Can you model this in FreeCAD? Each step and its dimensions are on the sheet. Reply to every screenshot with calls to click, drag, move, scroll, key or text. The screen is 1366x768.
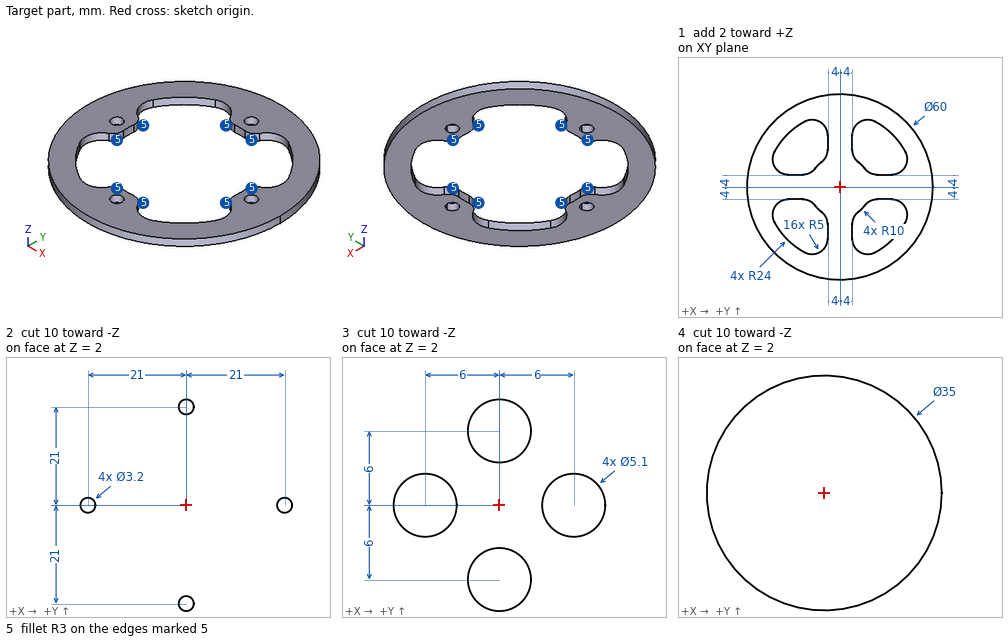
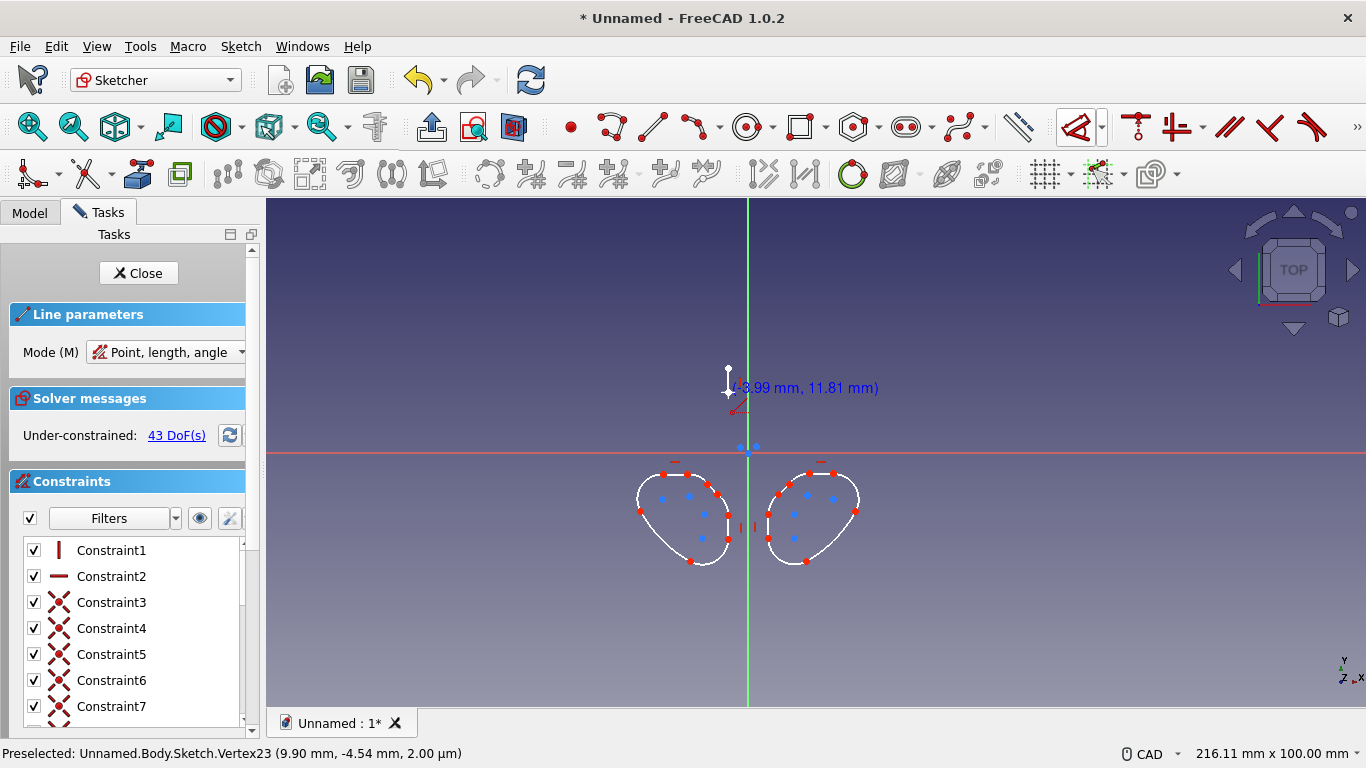
click(687, 433)
click(663, 433)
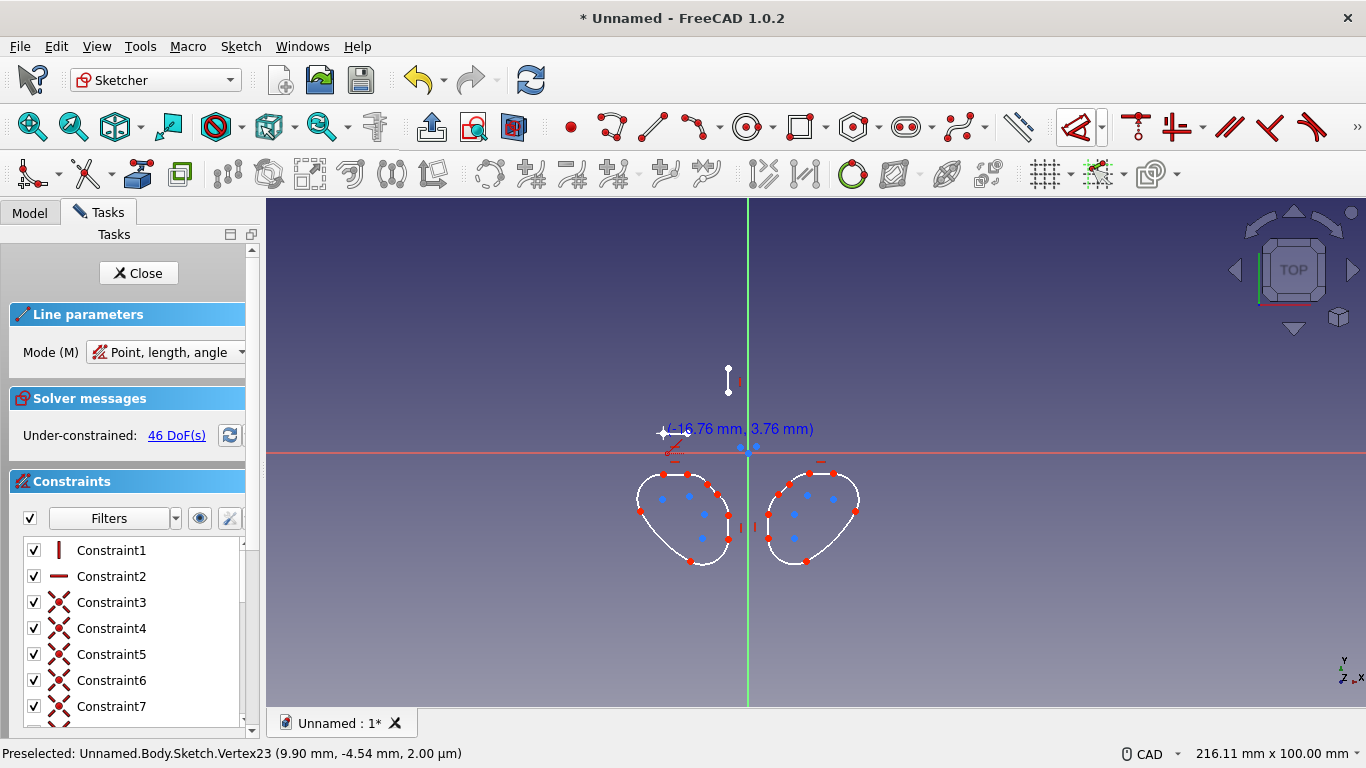
click(694, 128)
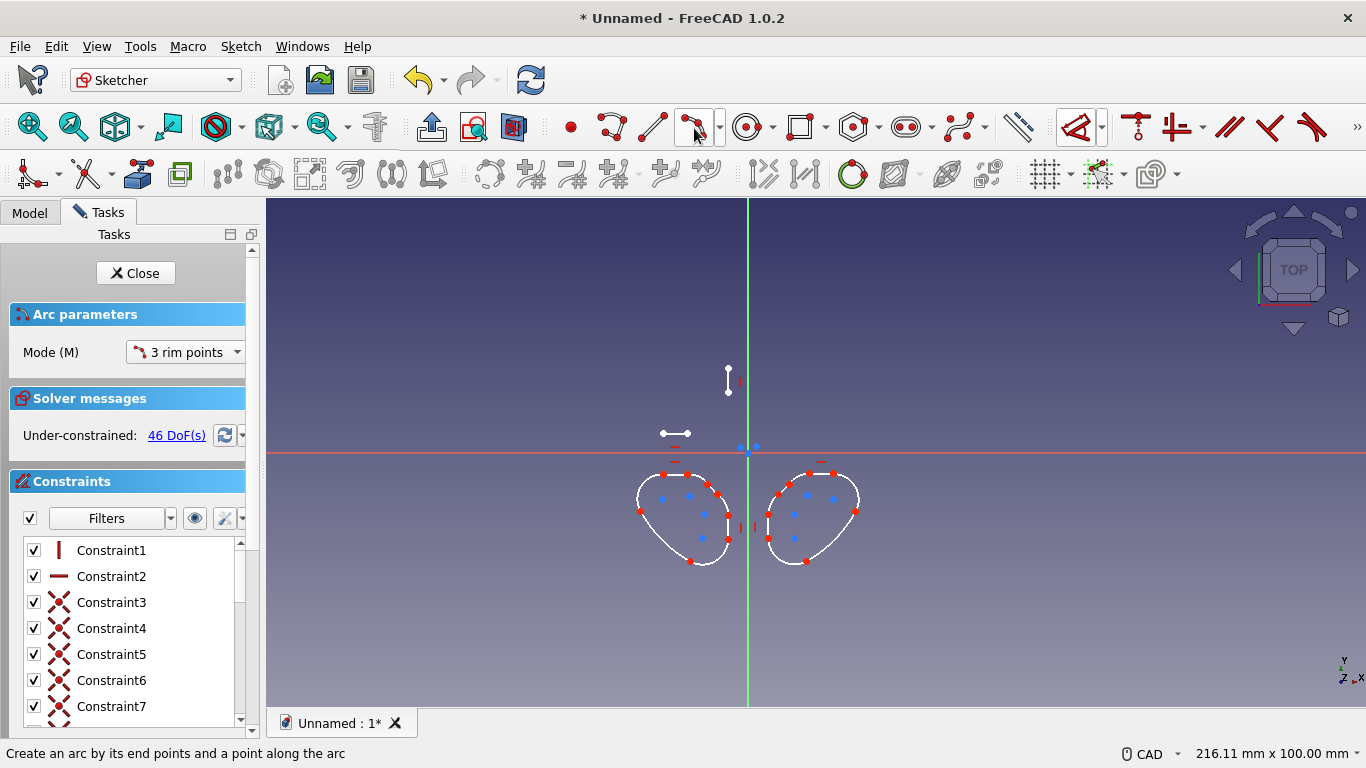
scroll(728, 392, up, 2)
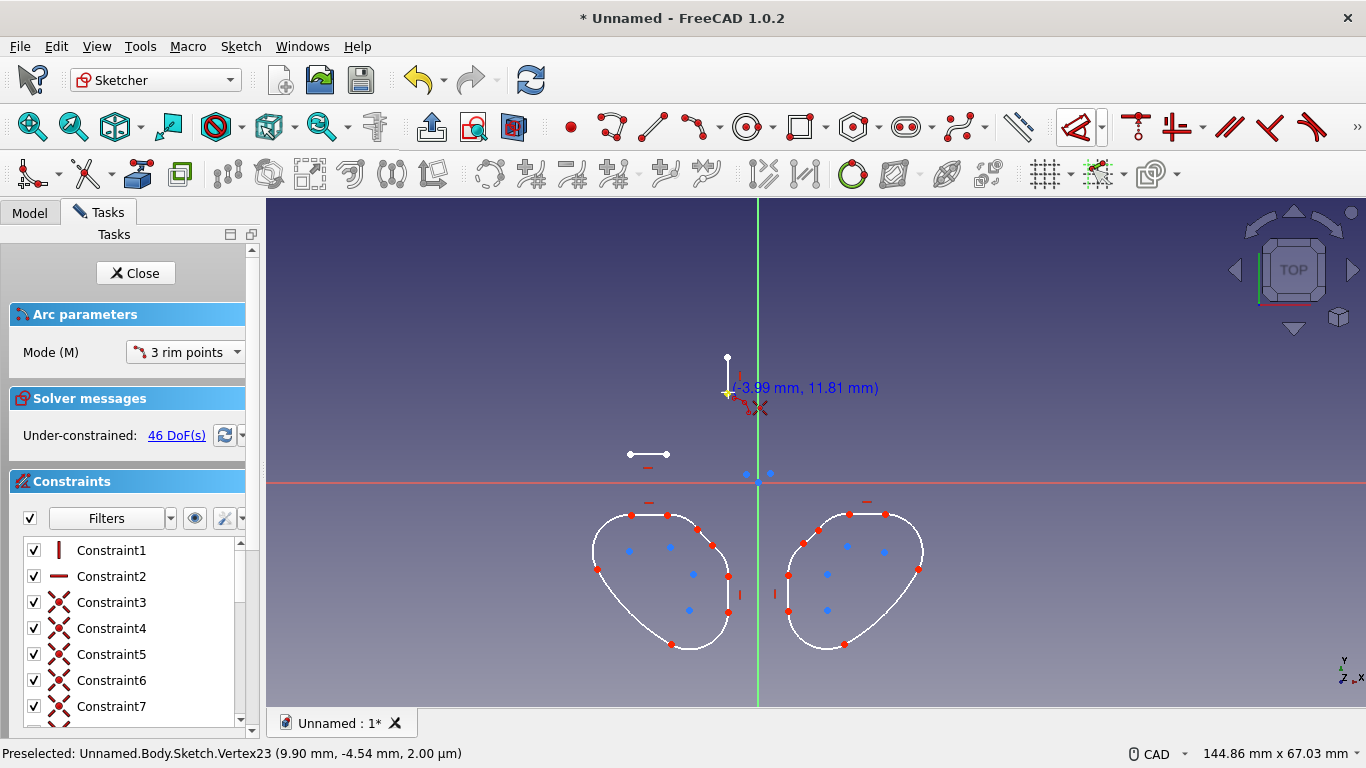
click(728, 393)
click(712, 422)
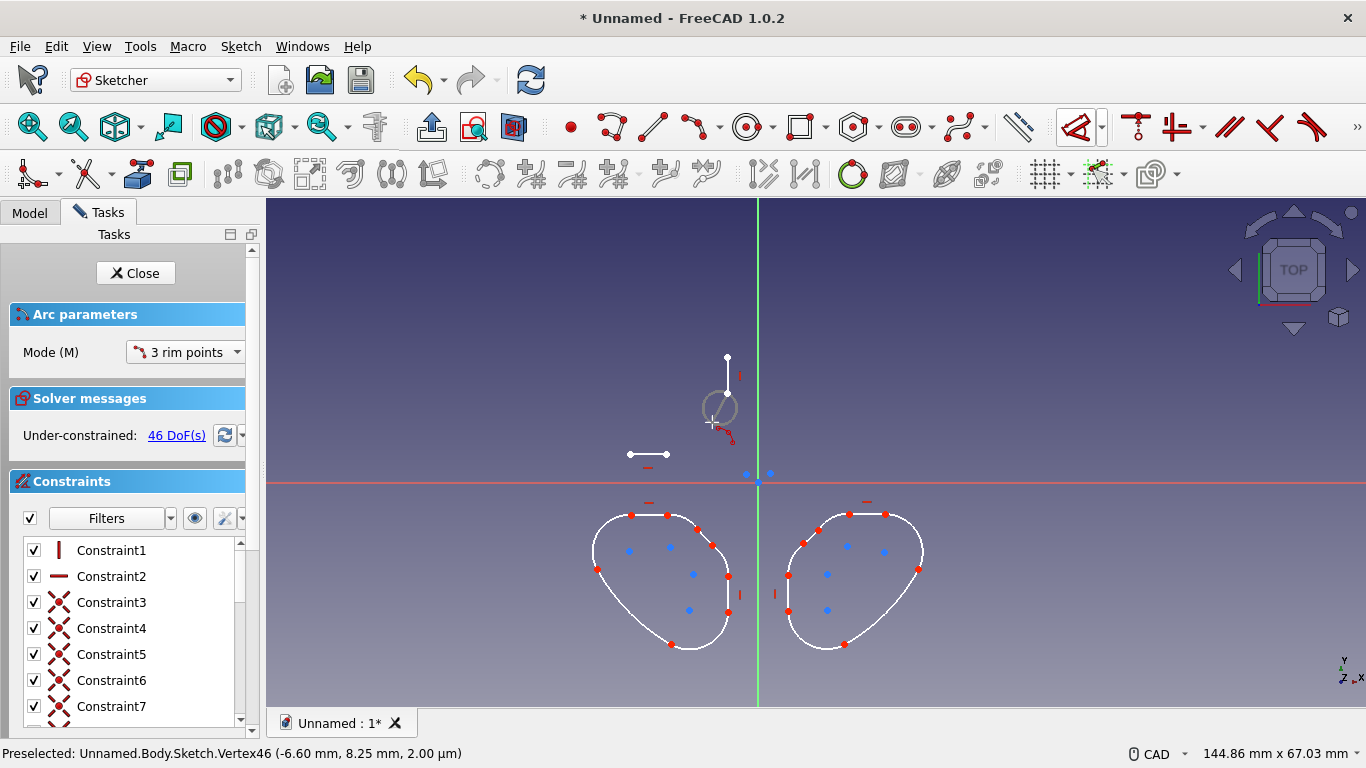
scroll(724, 409, up, 7)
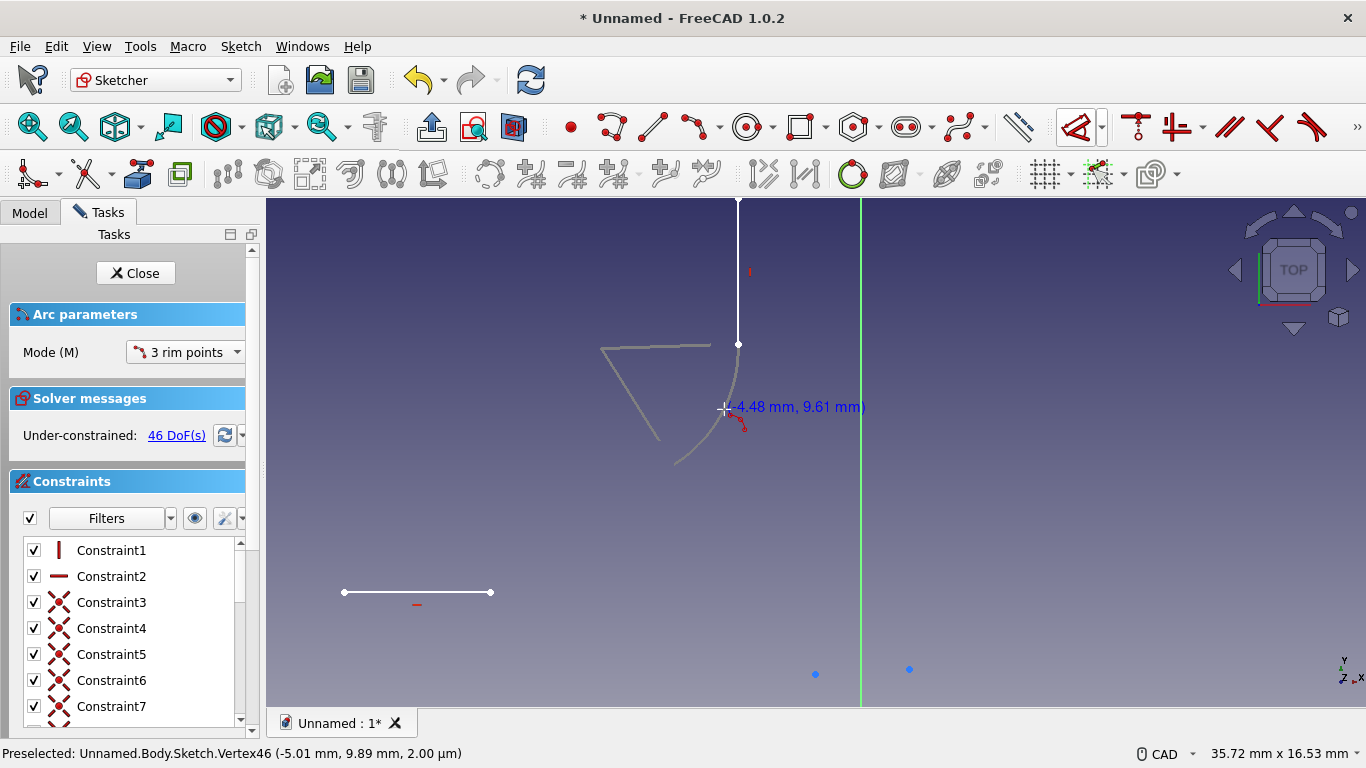
click(721, 407)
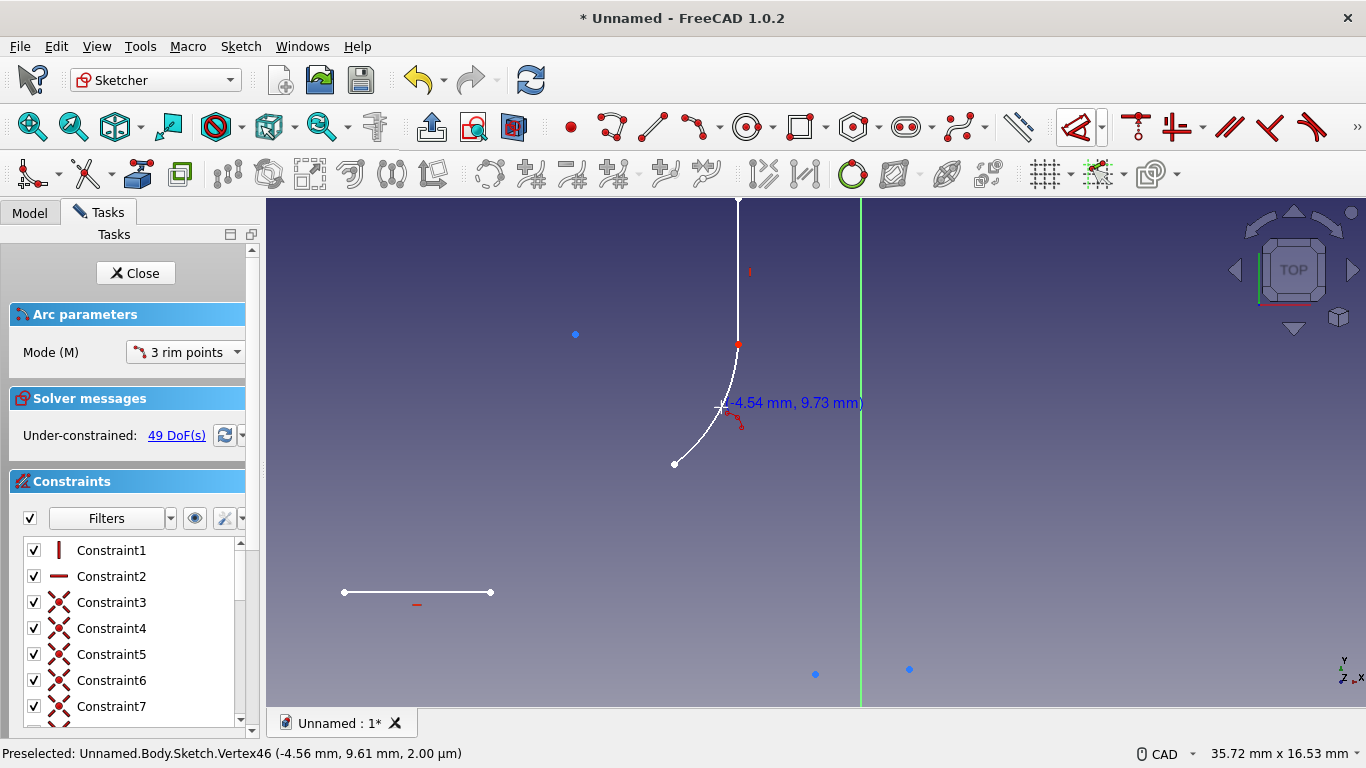
scroll(725, 402, down, 9)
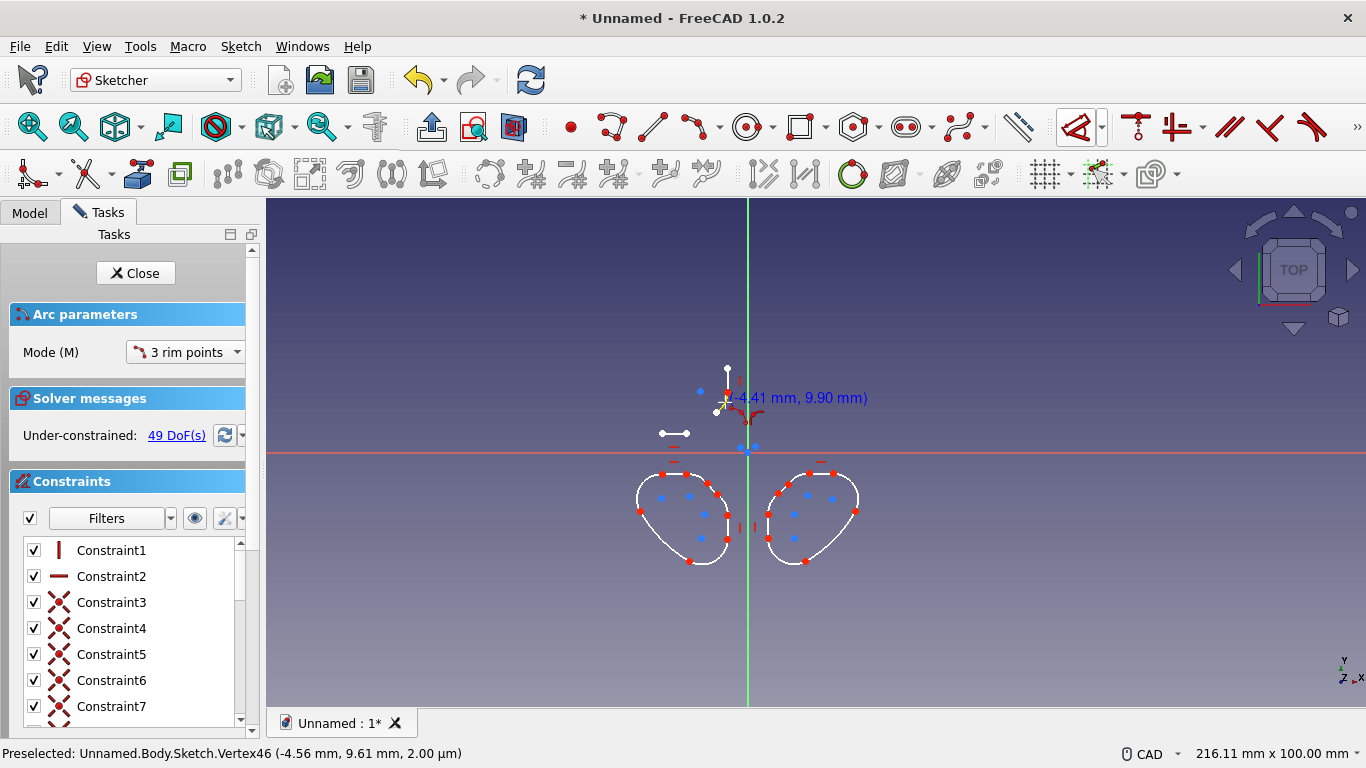
click(717, 413)
click(707, 422)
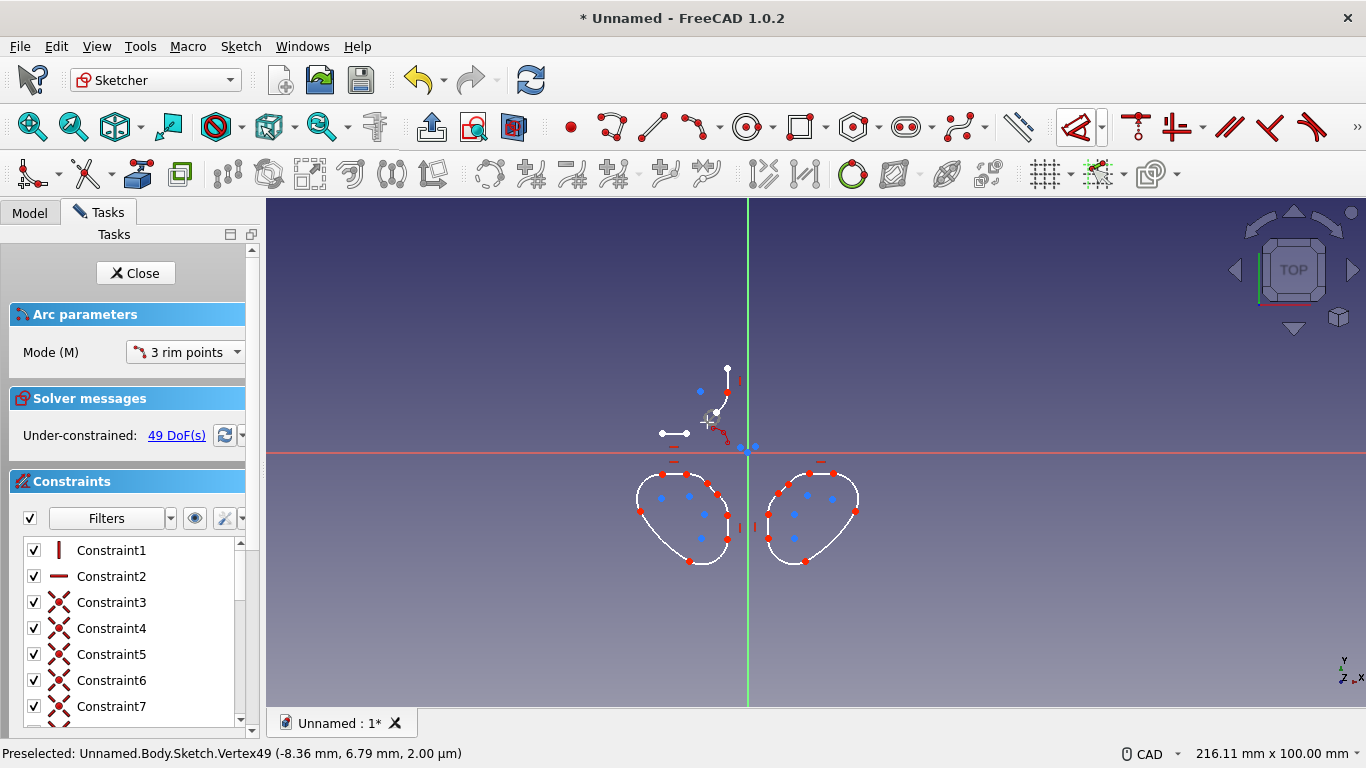
scroll(712, 417, up, 18)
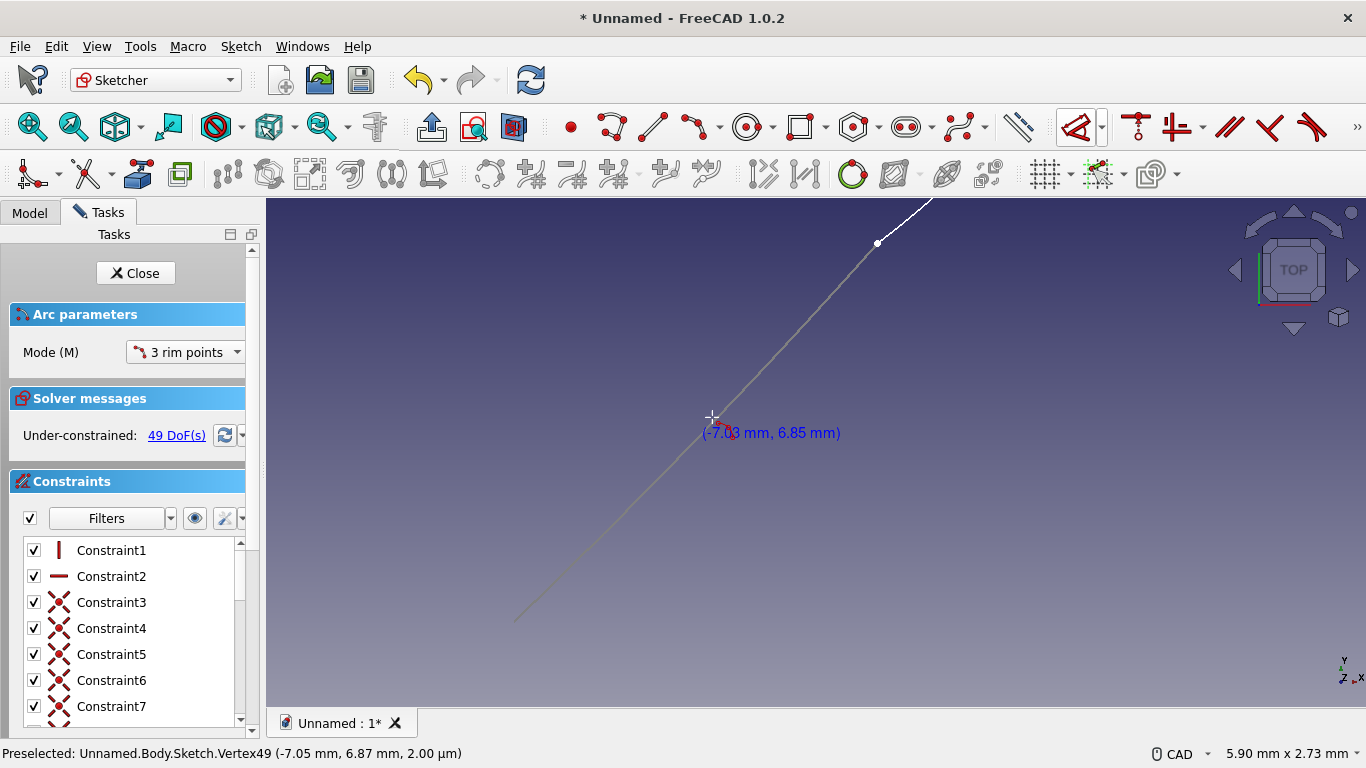
click(691, 397)